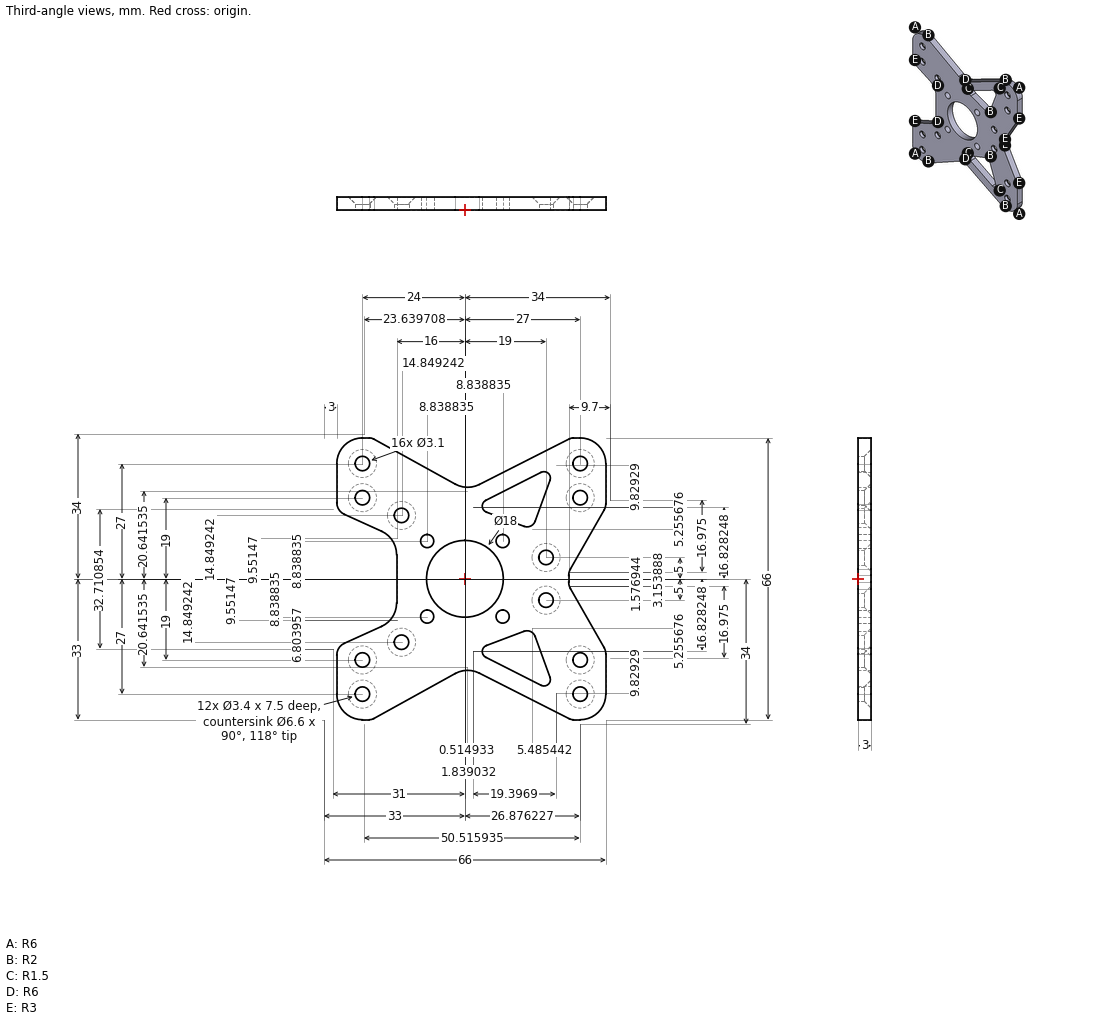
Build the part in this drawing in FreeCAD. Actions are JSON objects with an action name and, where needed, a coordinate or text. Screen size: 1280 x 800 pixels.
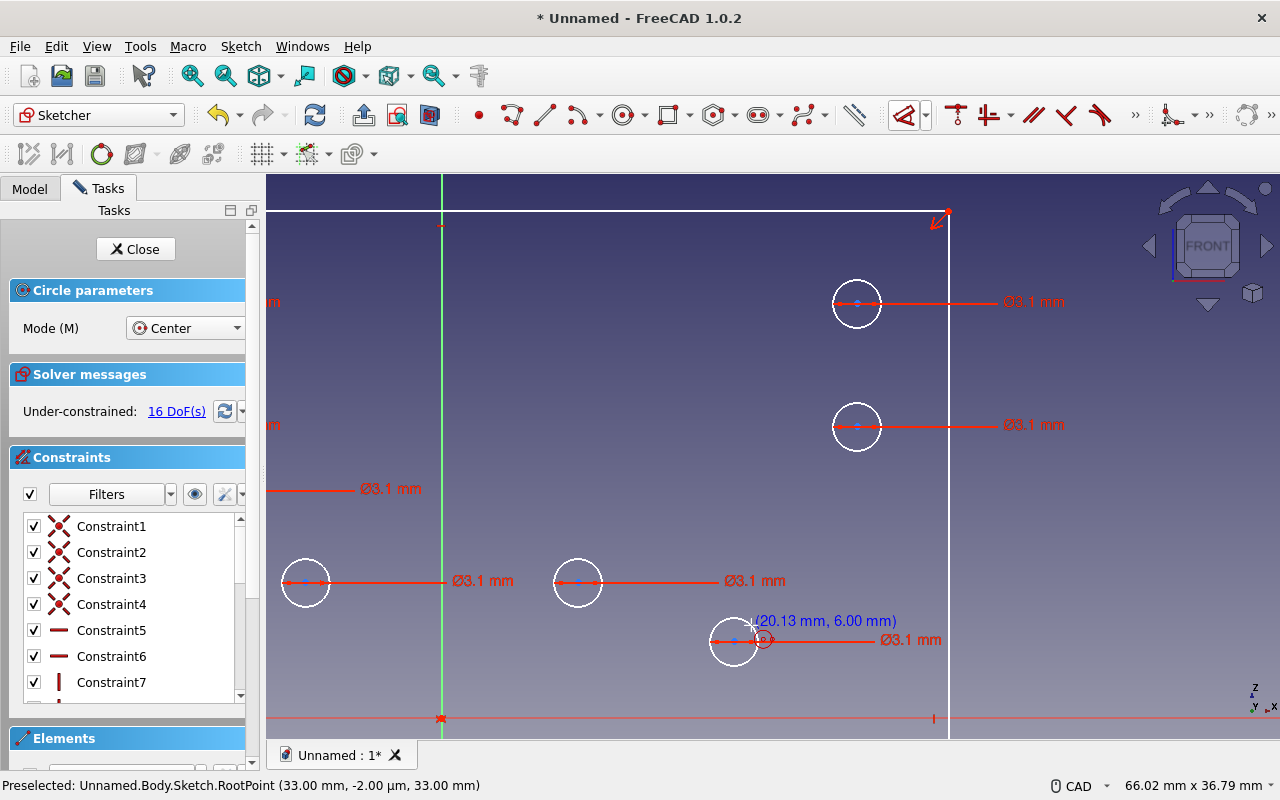
{"action": "scroll", "coordinate": [857, 304], "scroll_direction": "down", "scroll_amount": 5}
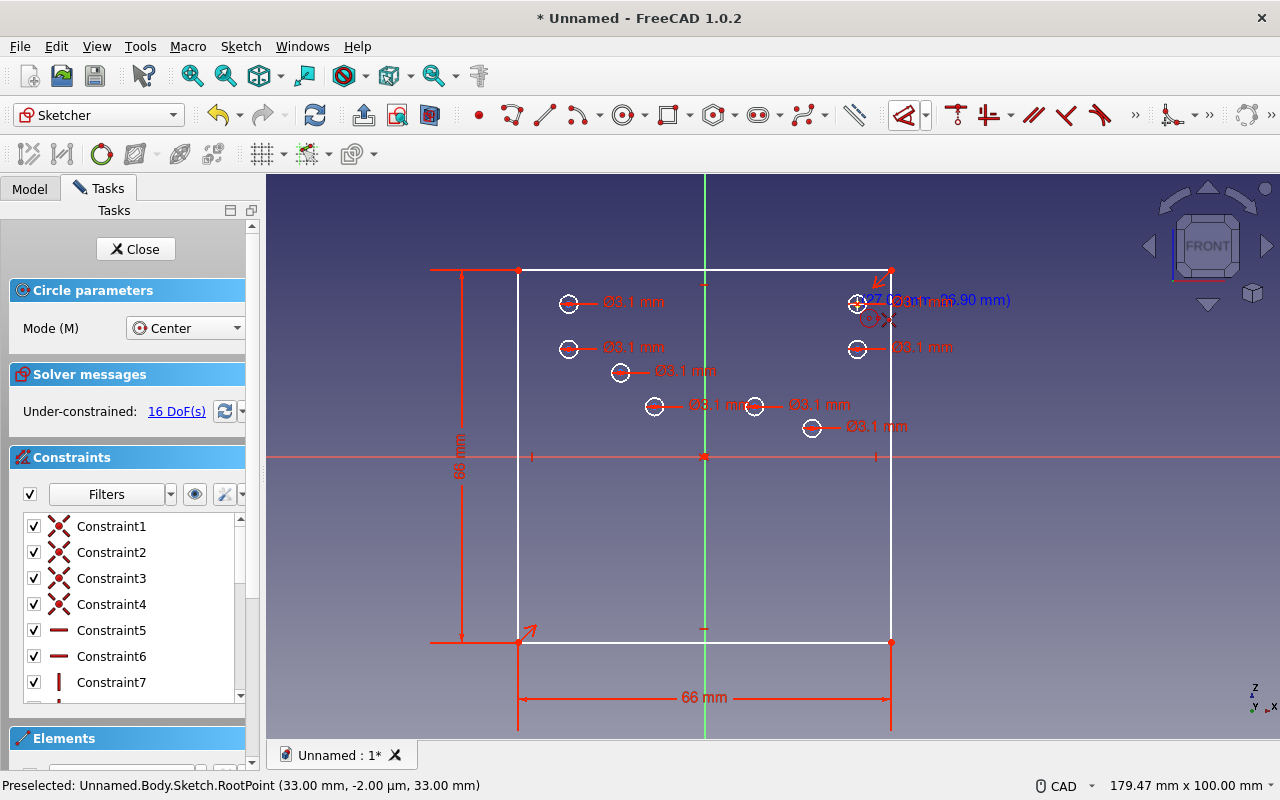
{"action": "left_click", "coordinate": [705, 456]}
{"action": "mouse_move", "coordinate": [741, 492]}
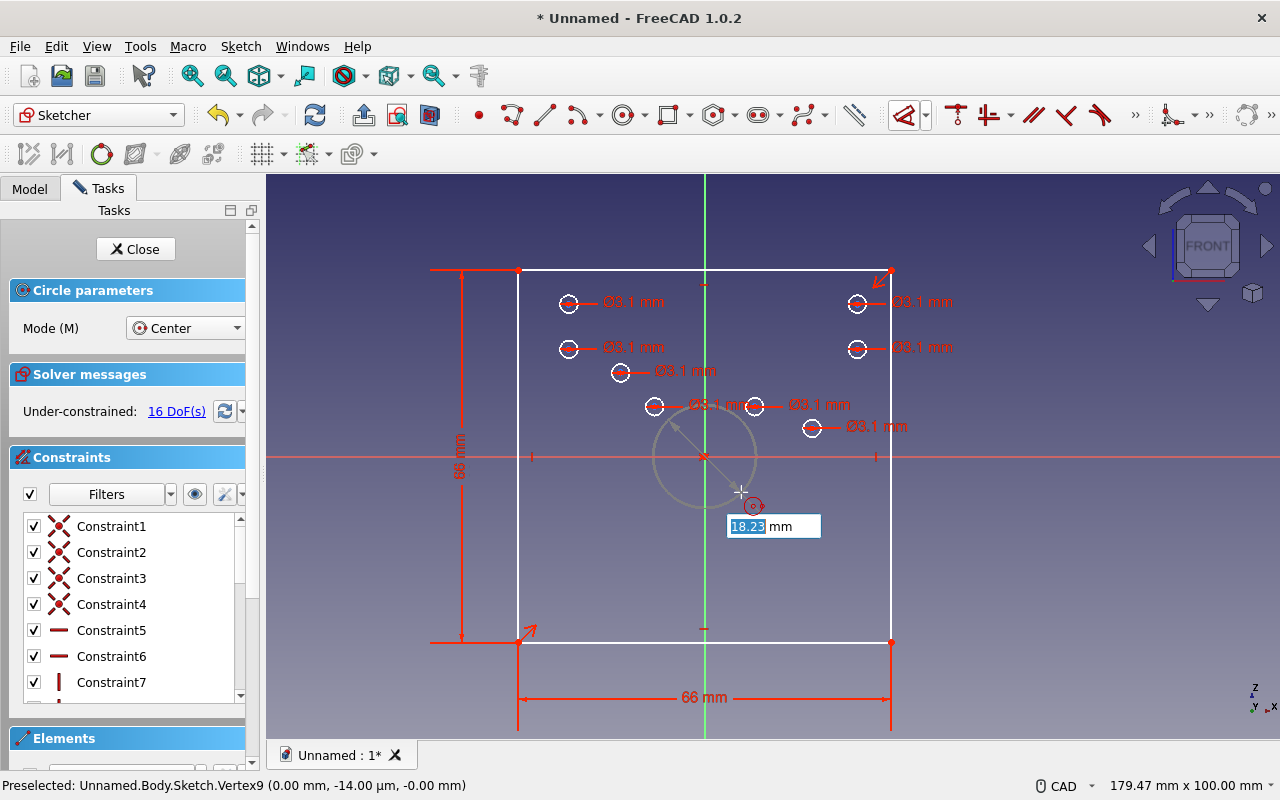
{"action": "type", "text": "18"}
{"action": "key", "text": "Return"}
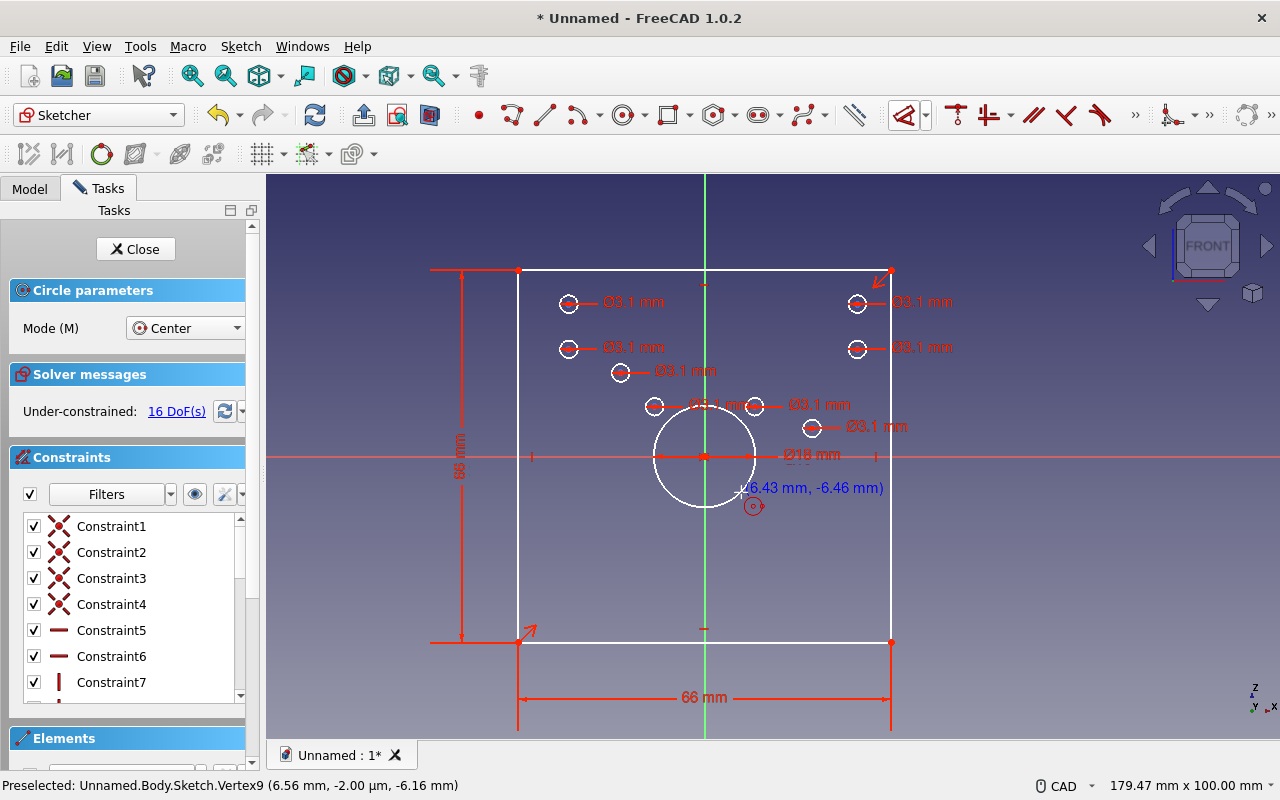
{"action": "scroll", "coordinate": [655, 506], "scroll_direction": "up", "scroll_amount": 5}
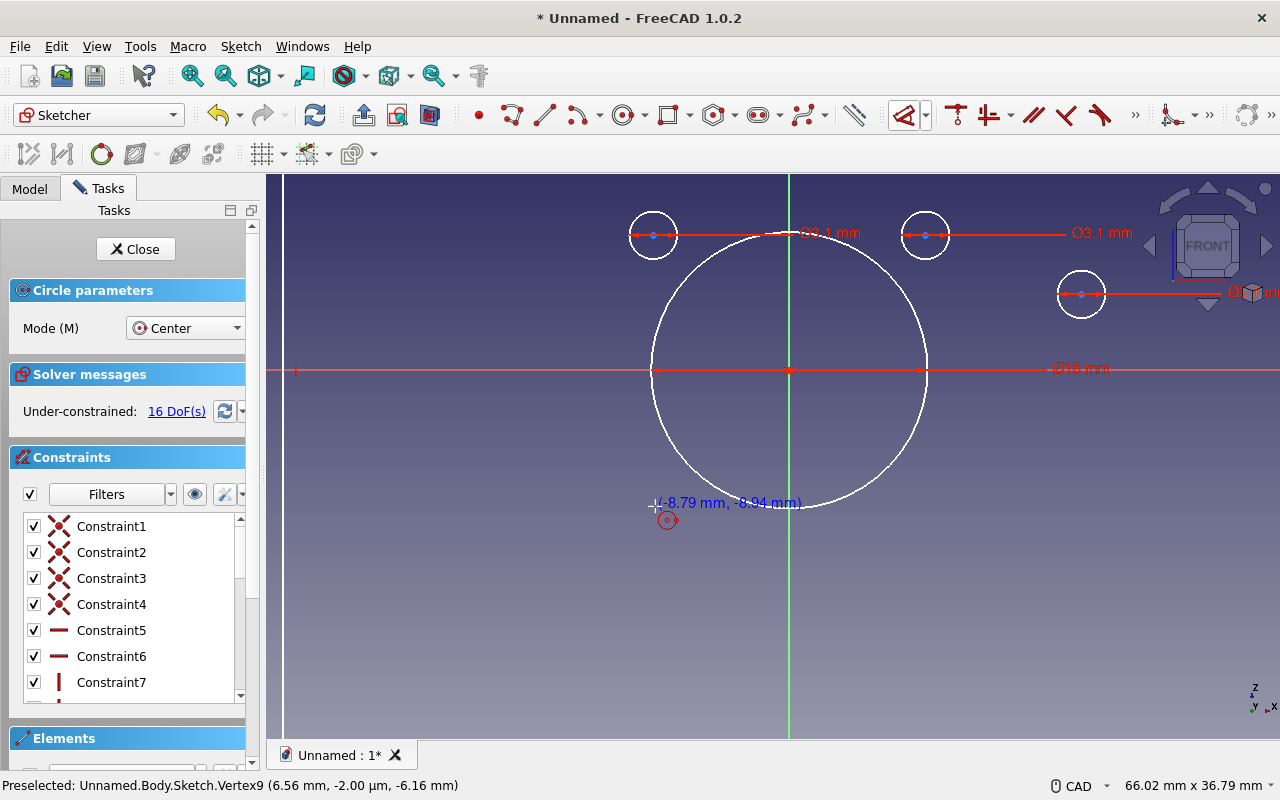
{"action": "left_click", "coordinate": [654, 506]}
{"action": "mouse_move", "coordinate": [670, 489]}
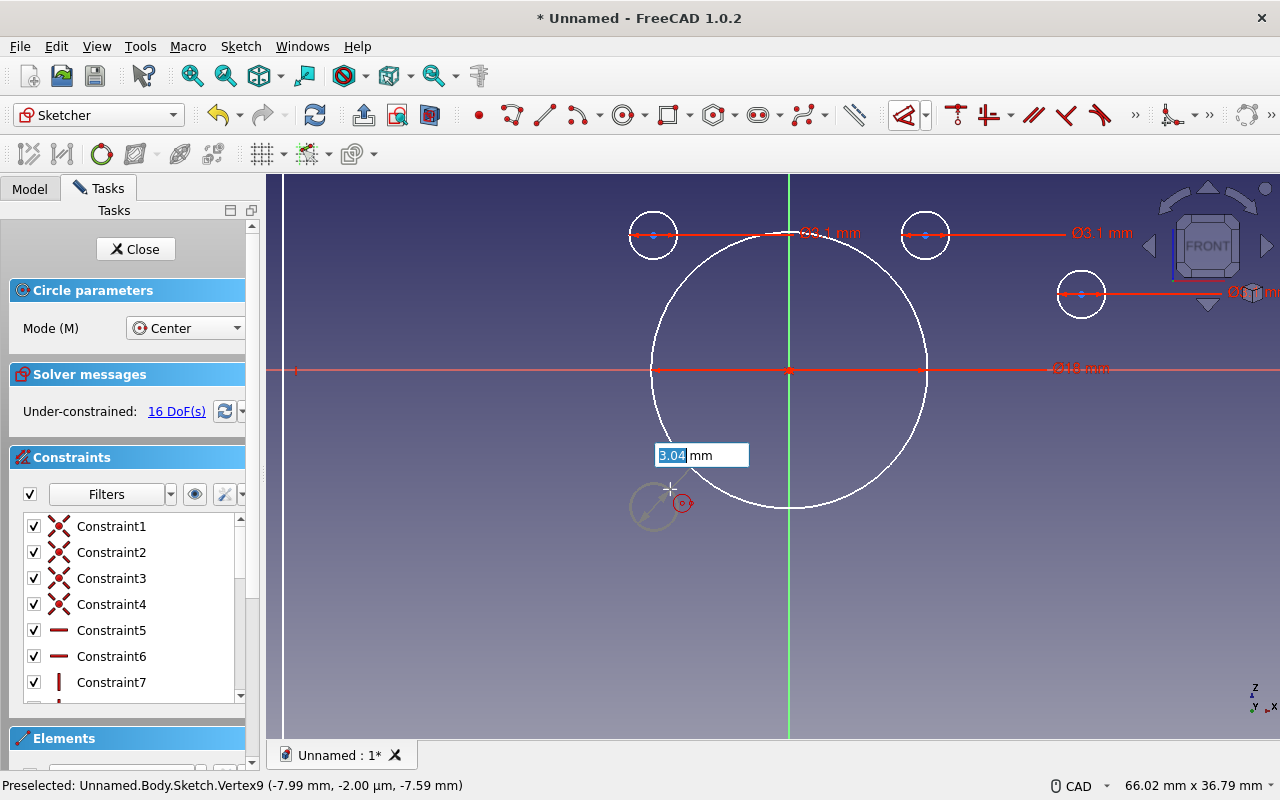
{"action": "type", "text": "3.1"}
{"action": "key", "text": "Return"}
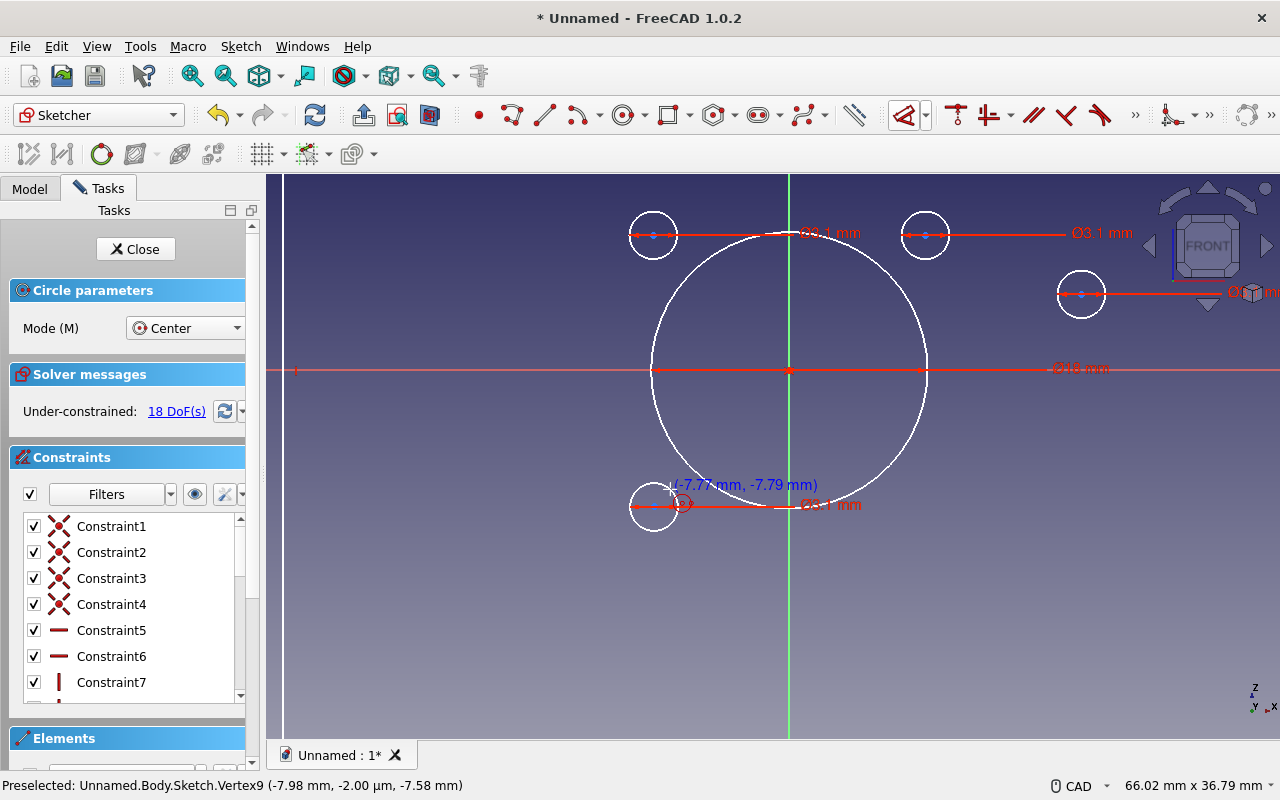
{"action": "left_click", "coordinate": [421, 662]}
{"action": "mouse_move", "coordinate": [438, 645]}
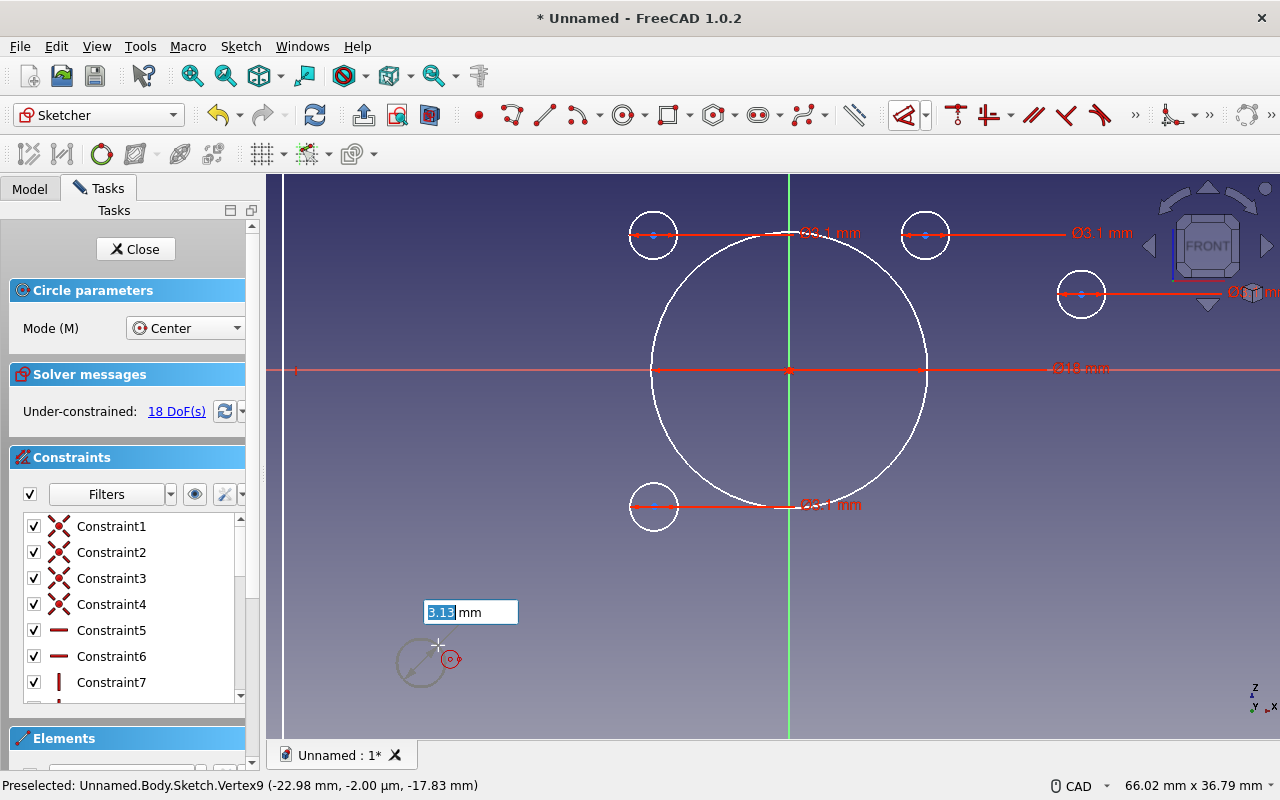
{"action": "type", "text": "3.1"}
{"action": "key", "text": "Return"}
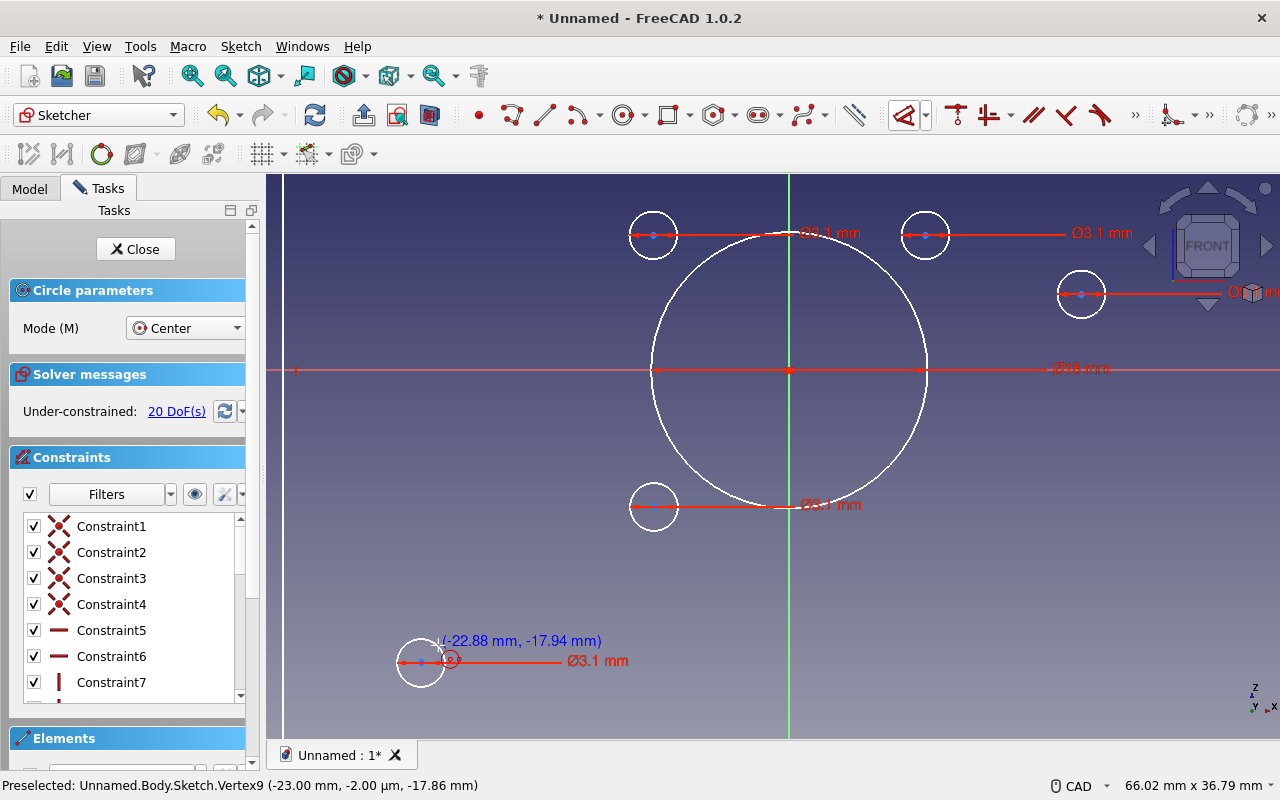
{"action": "left_click", "coordinate": [561, 598]}
{"action": "mouse_move", "coordinate": [578, 582]}